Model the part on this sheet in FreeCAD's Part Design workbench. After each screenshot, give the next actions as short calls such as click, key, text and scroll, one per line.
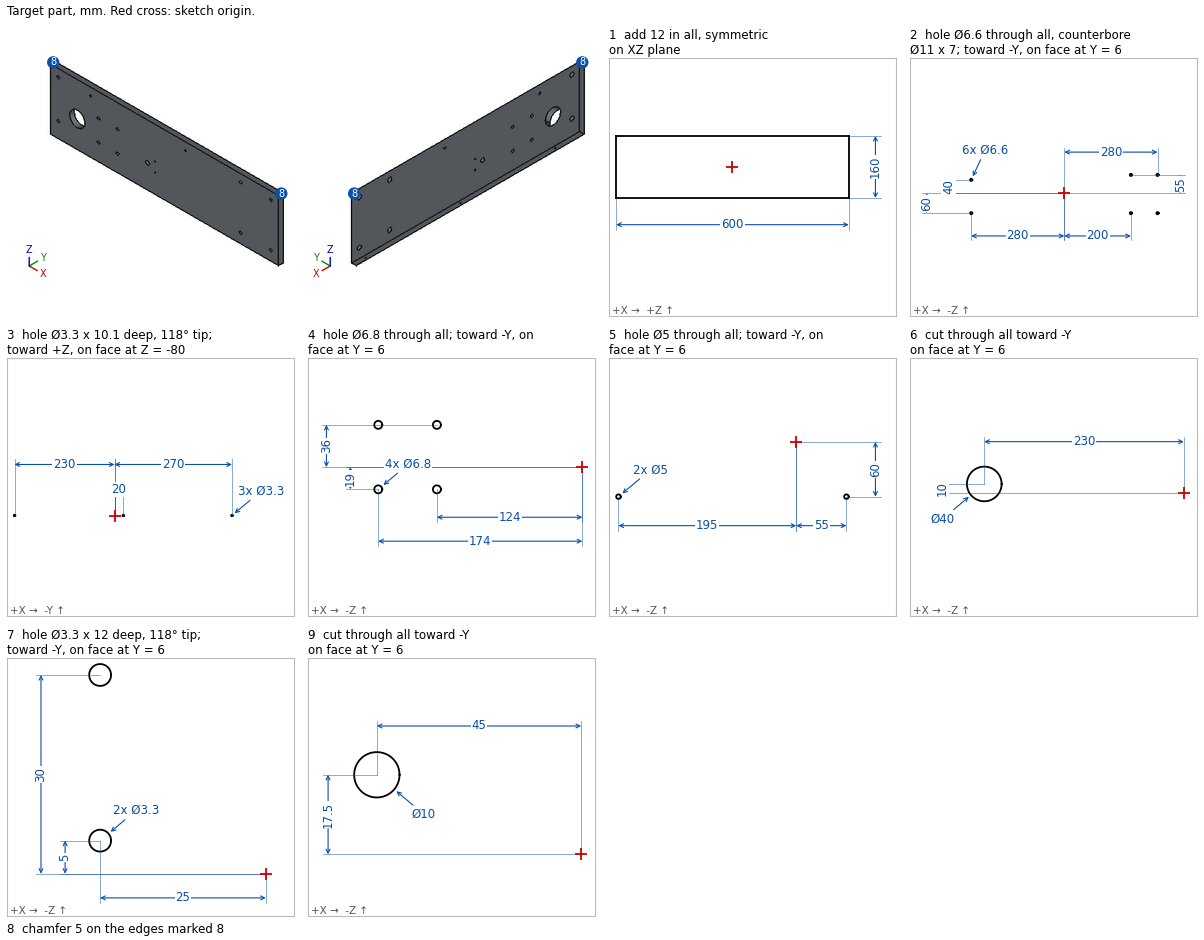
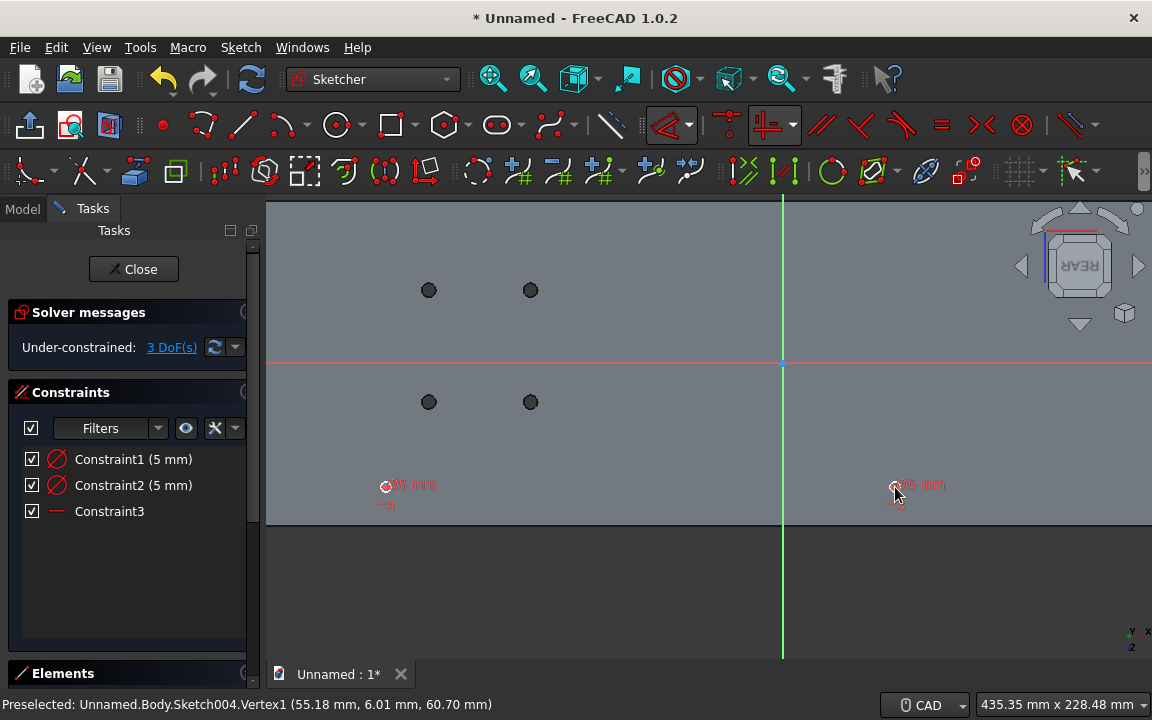
click(692, 126)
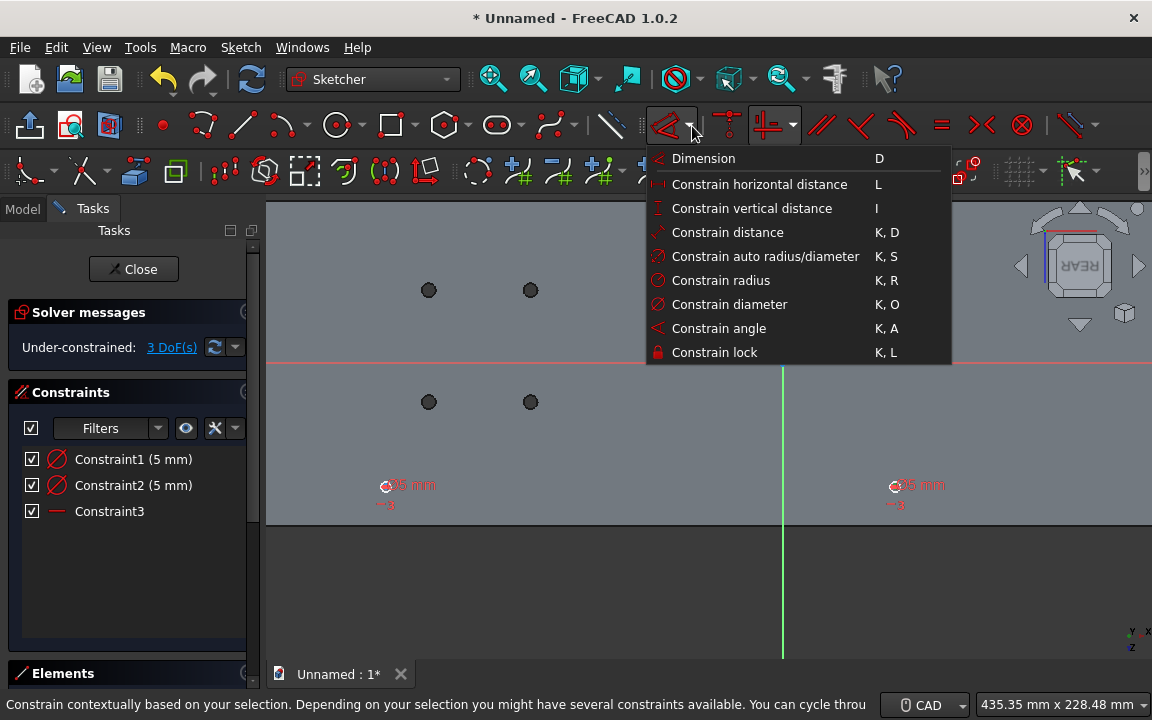
click(799, 184)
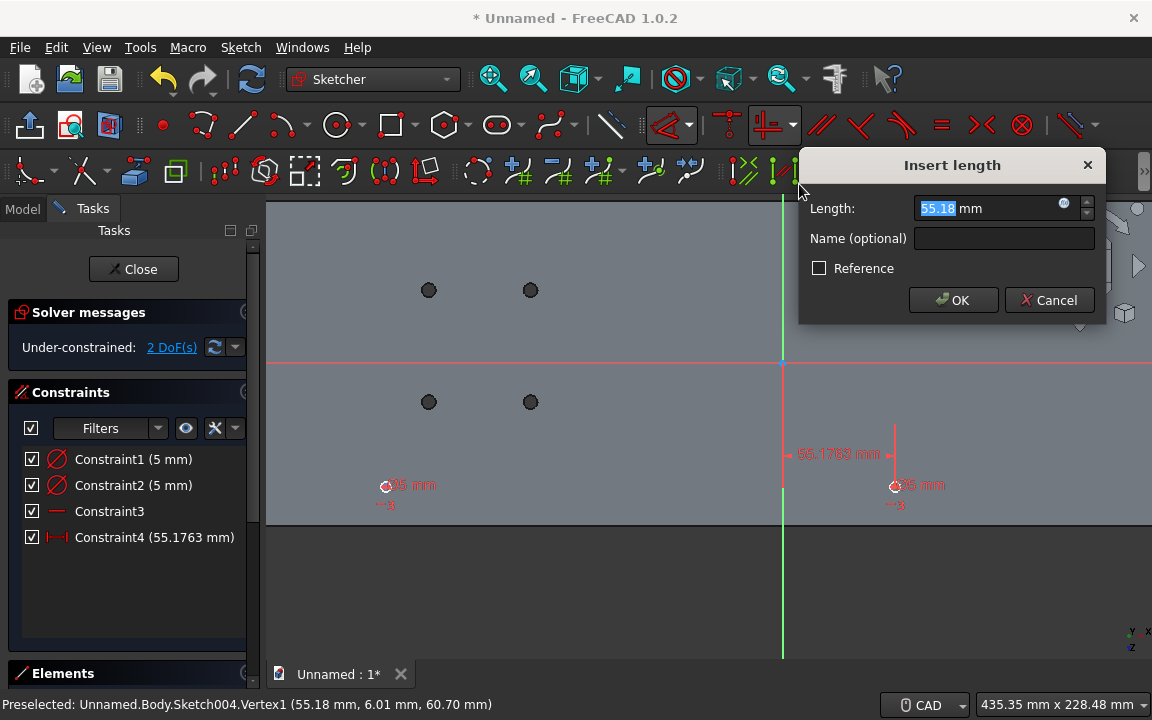
text(55)
key(Return)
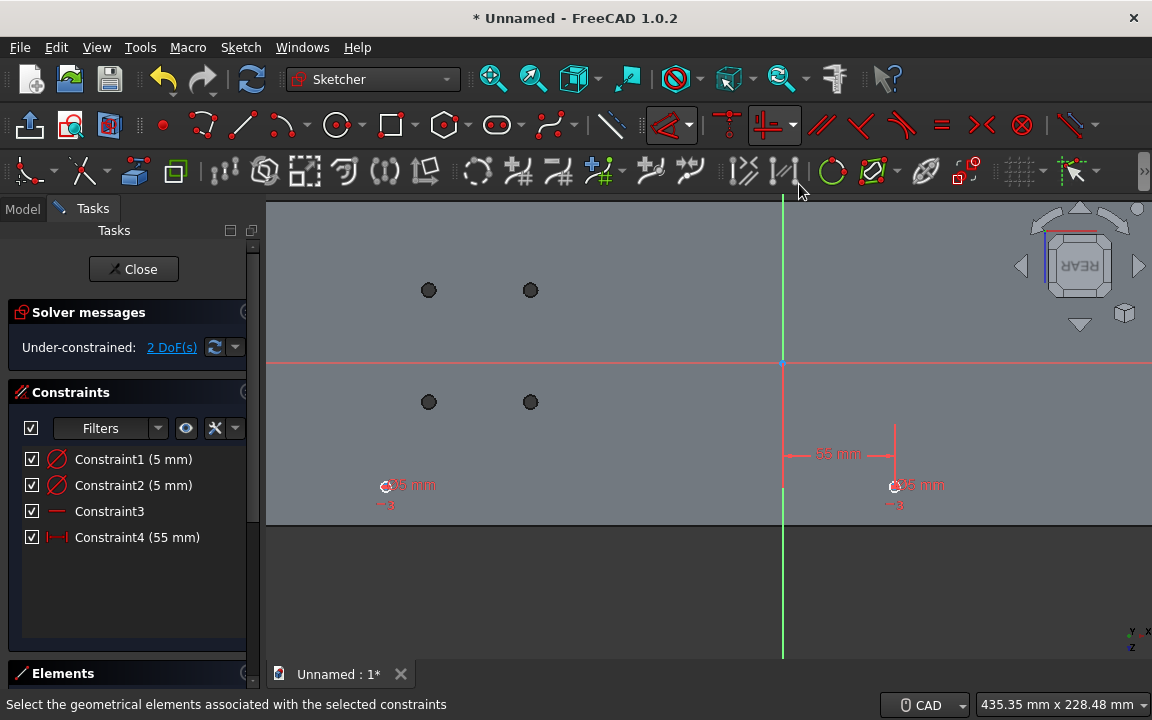
click(895, 487)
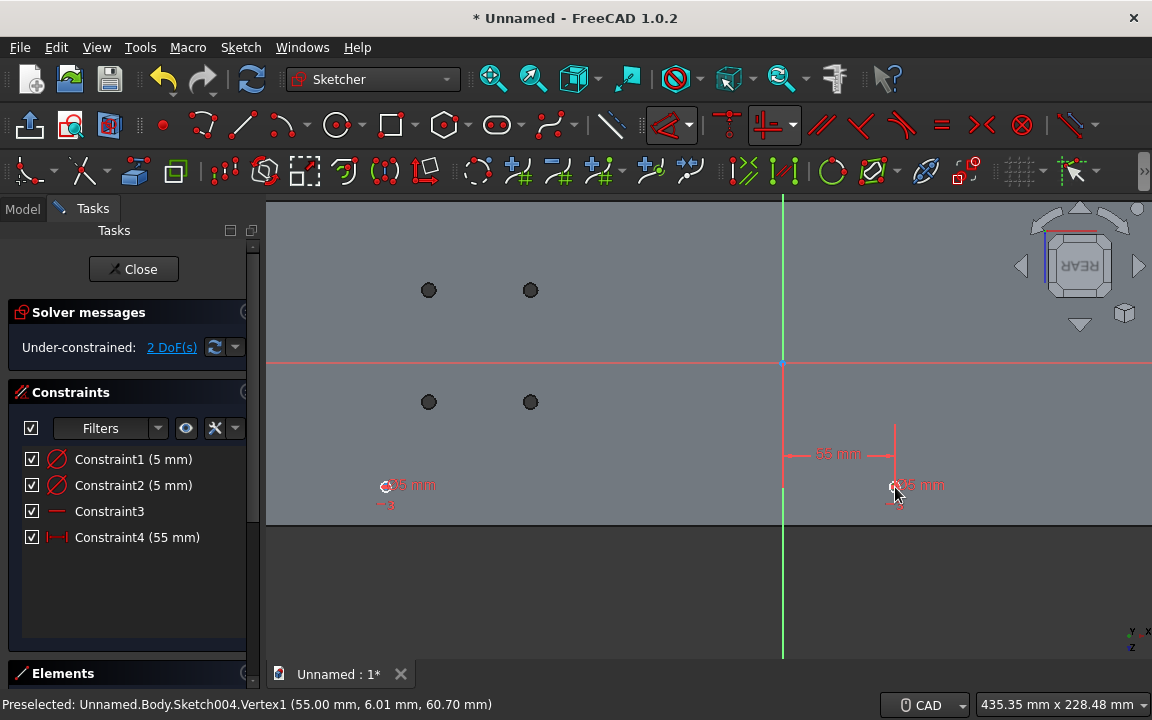
key(i)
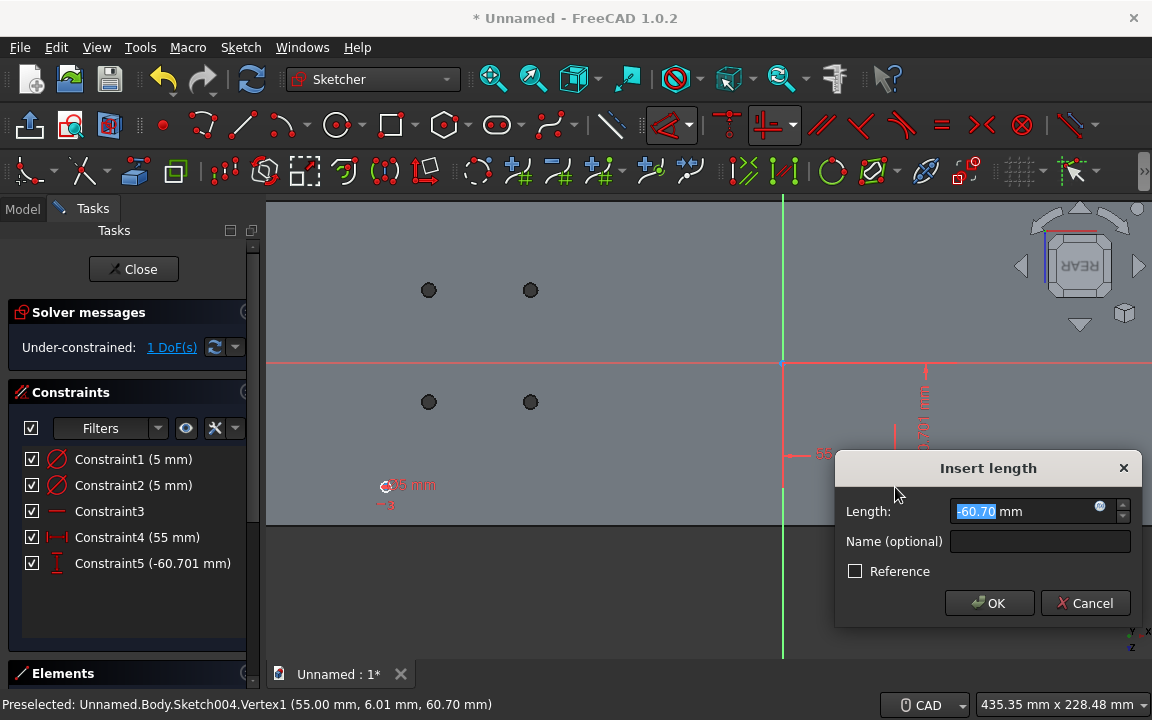
text(-60)
key(Return)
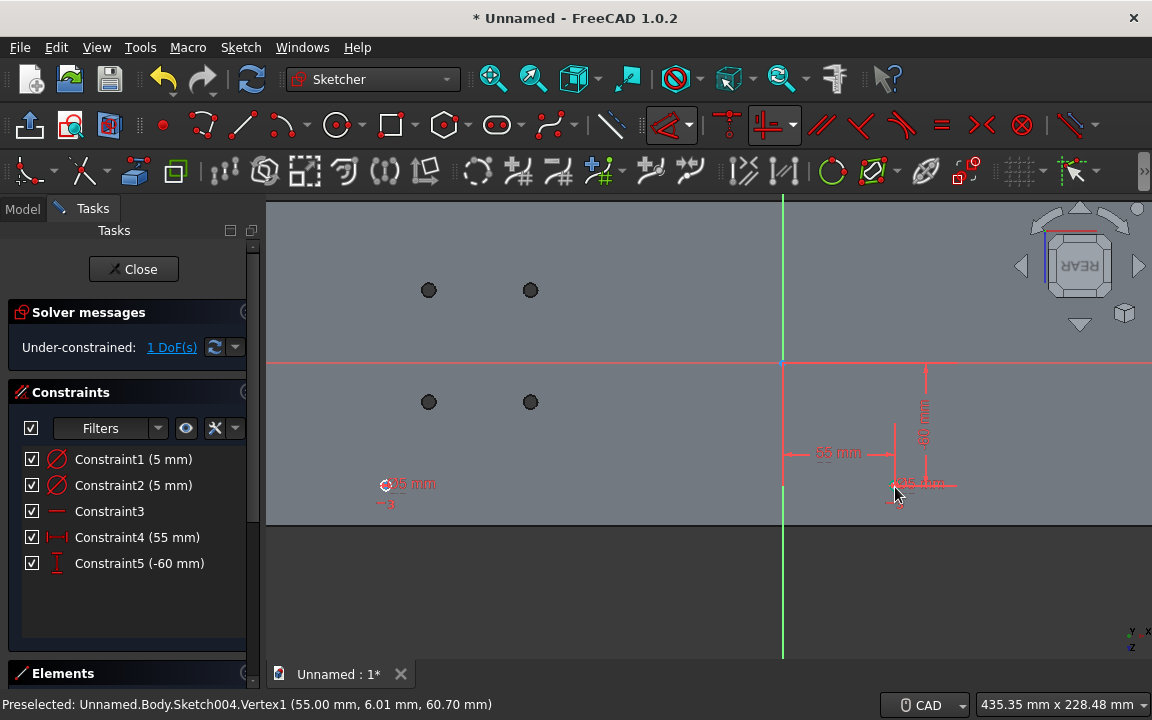
click(386, 486)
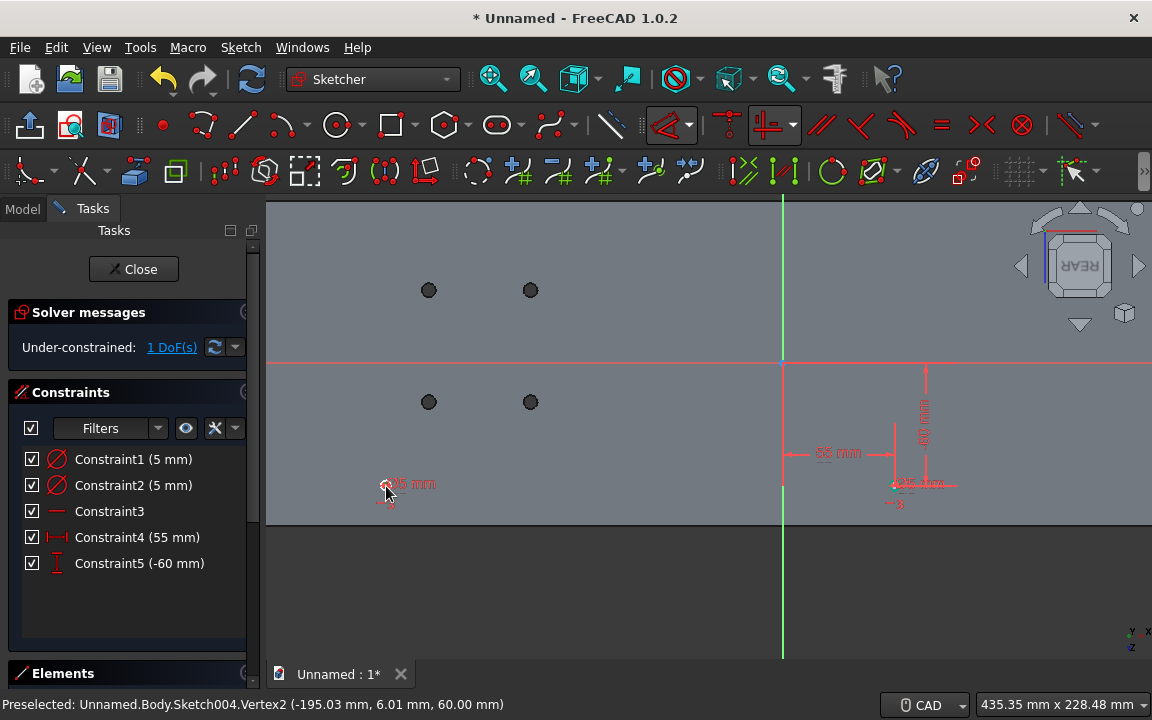
click(692, 126)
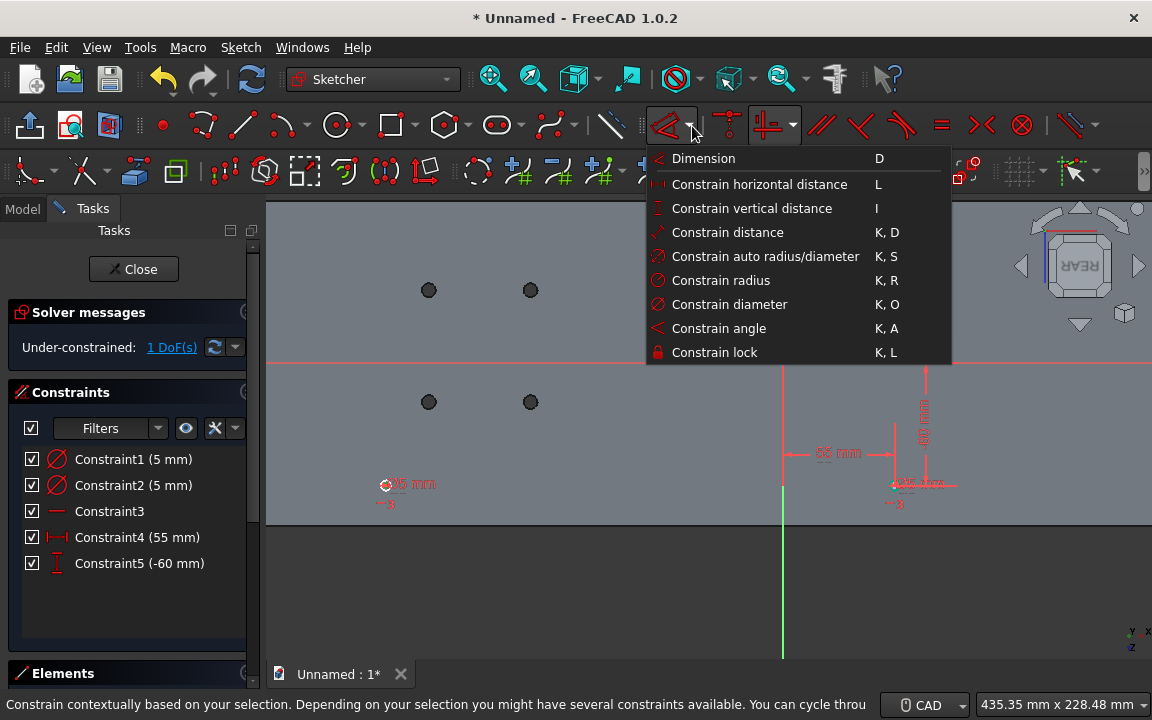
click(799, 184)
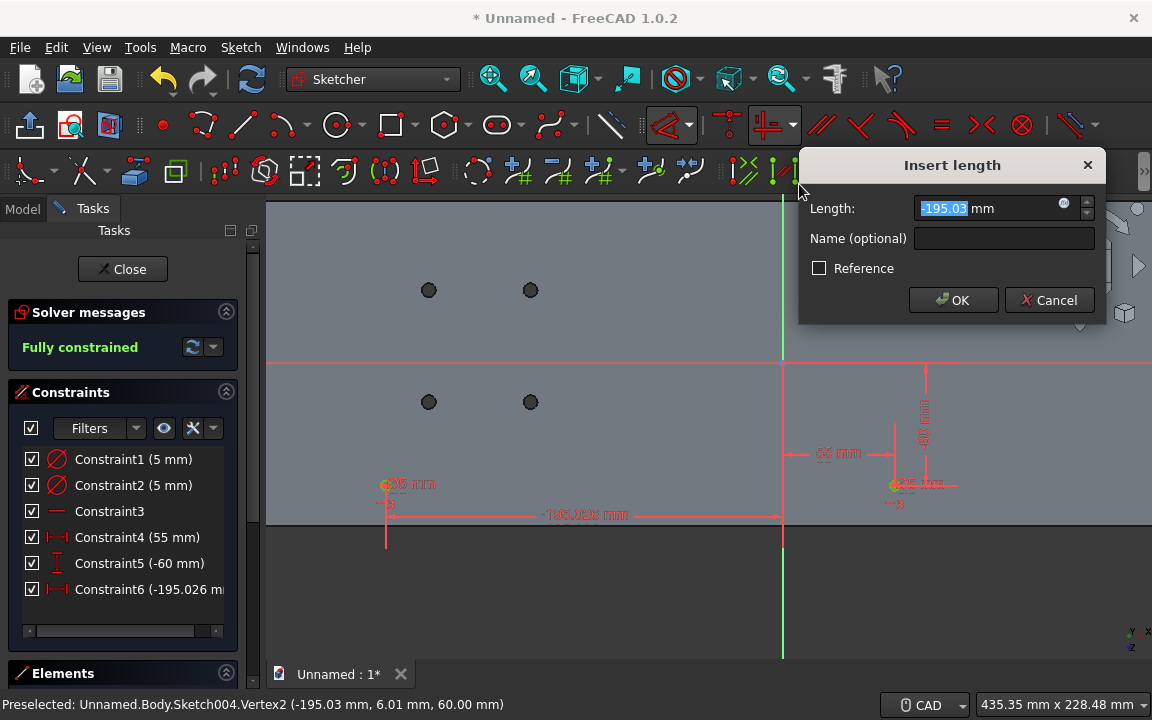
text(-195)
key(Return)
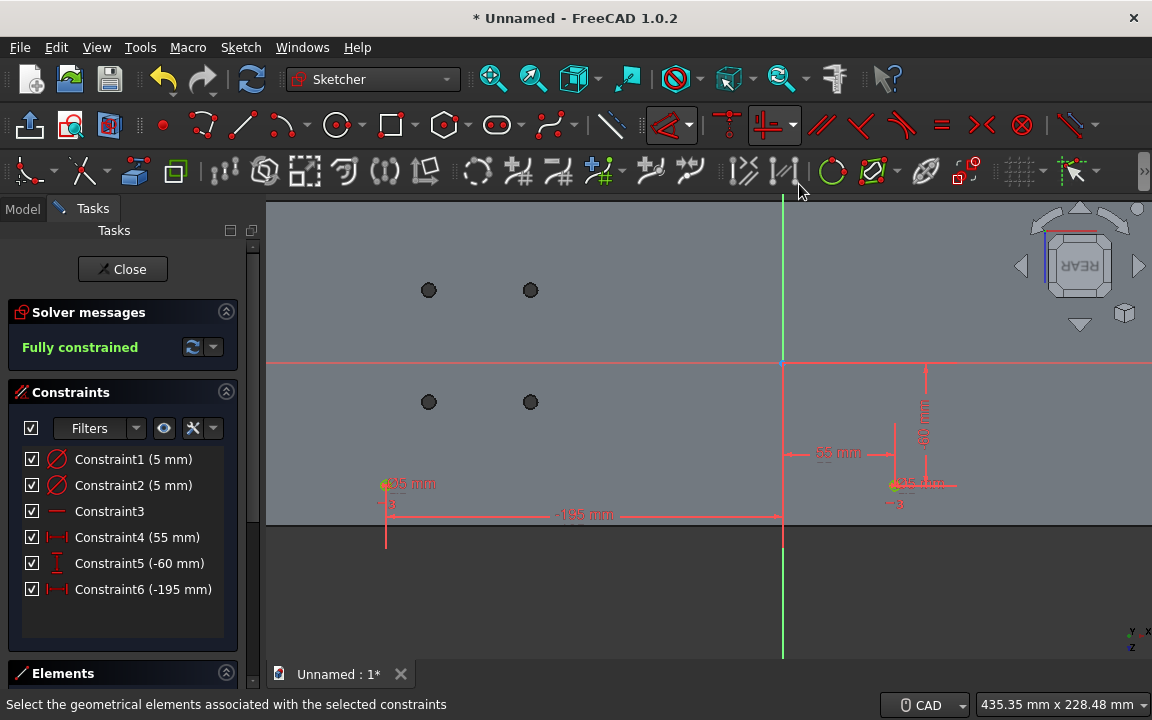
click(123, 269)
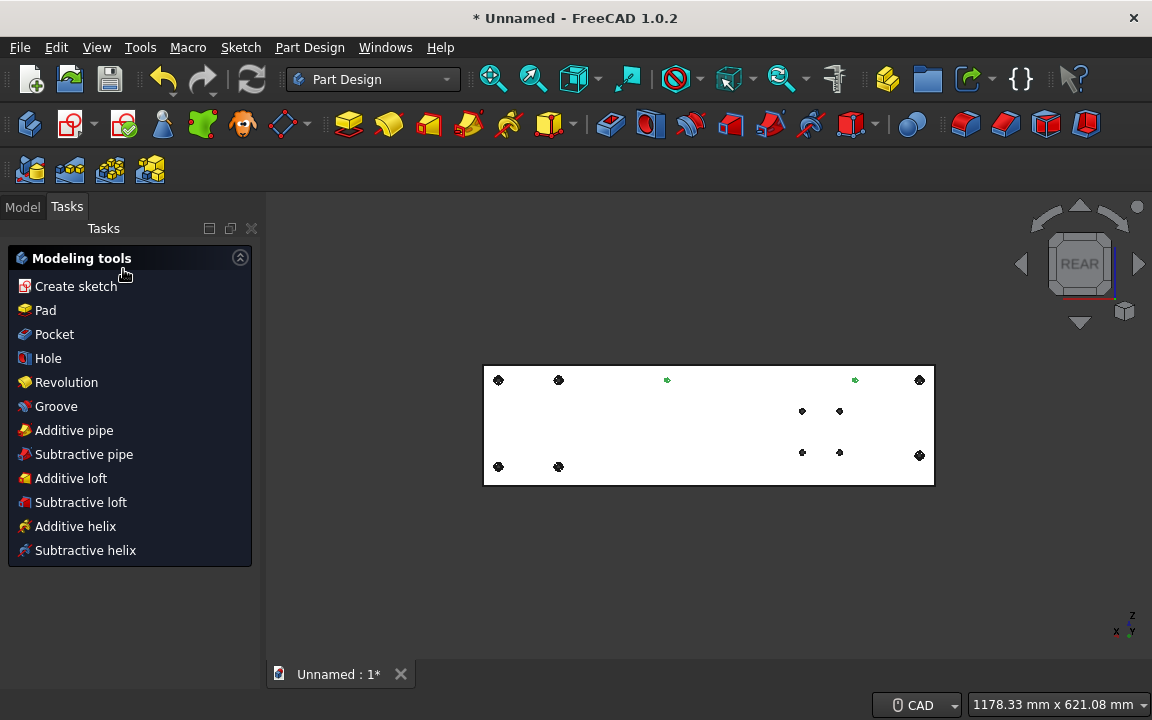
click(652, 124)